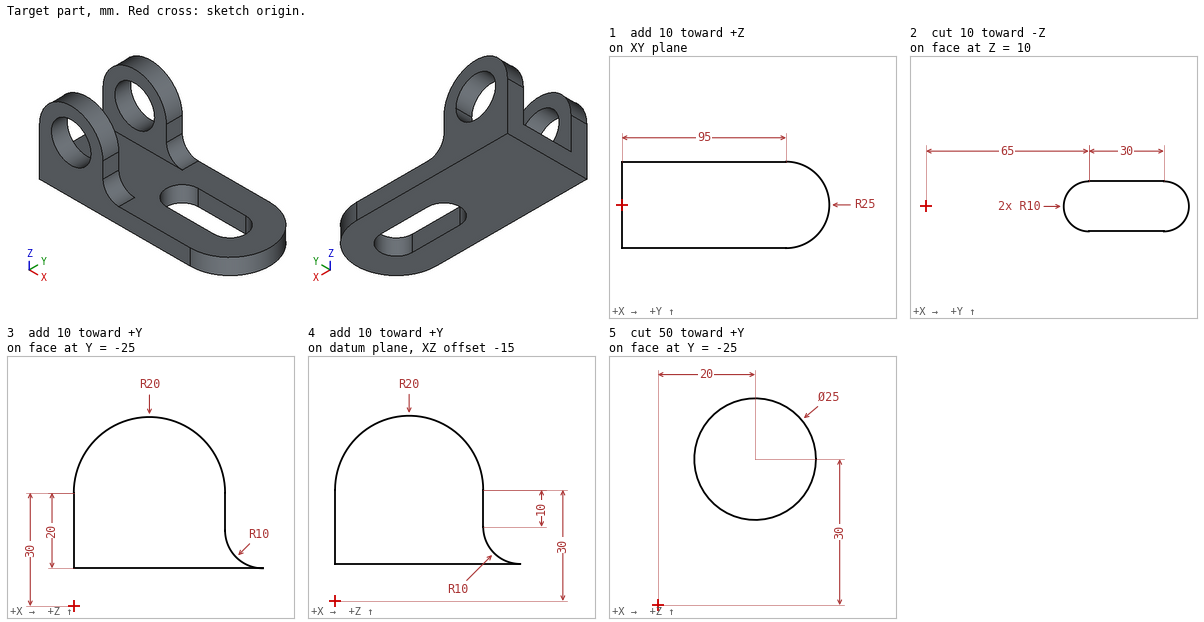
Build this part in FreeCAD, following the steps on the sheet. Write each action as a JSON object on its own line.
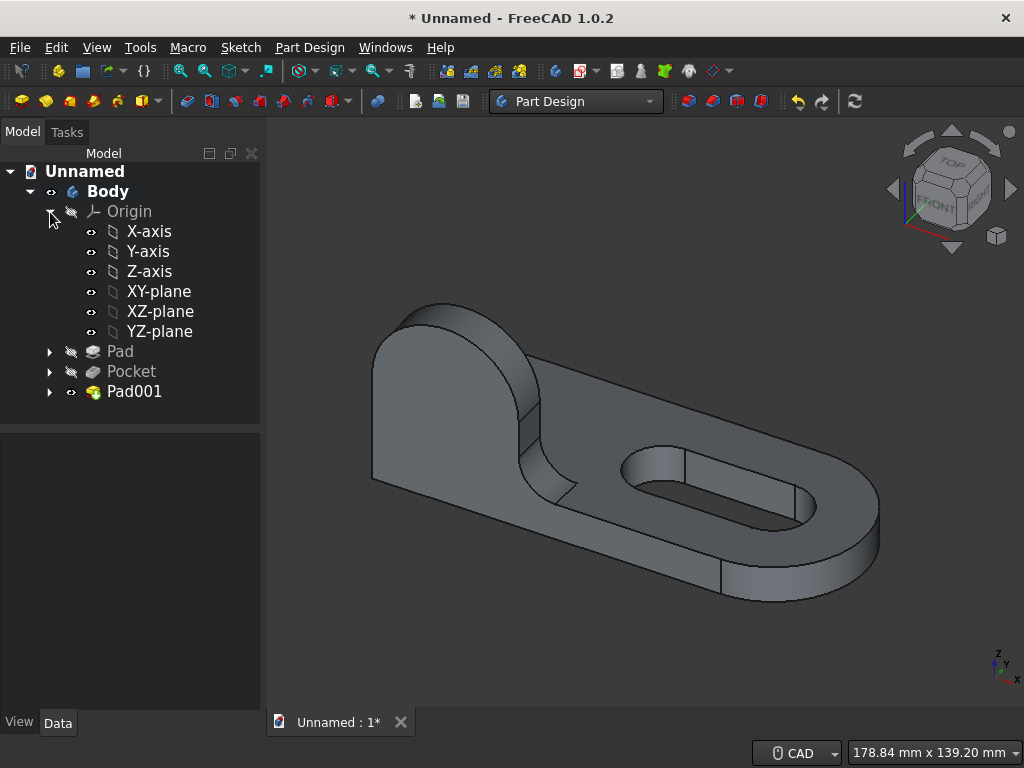
{"action": "left_click", "coordinate": [136, 312]}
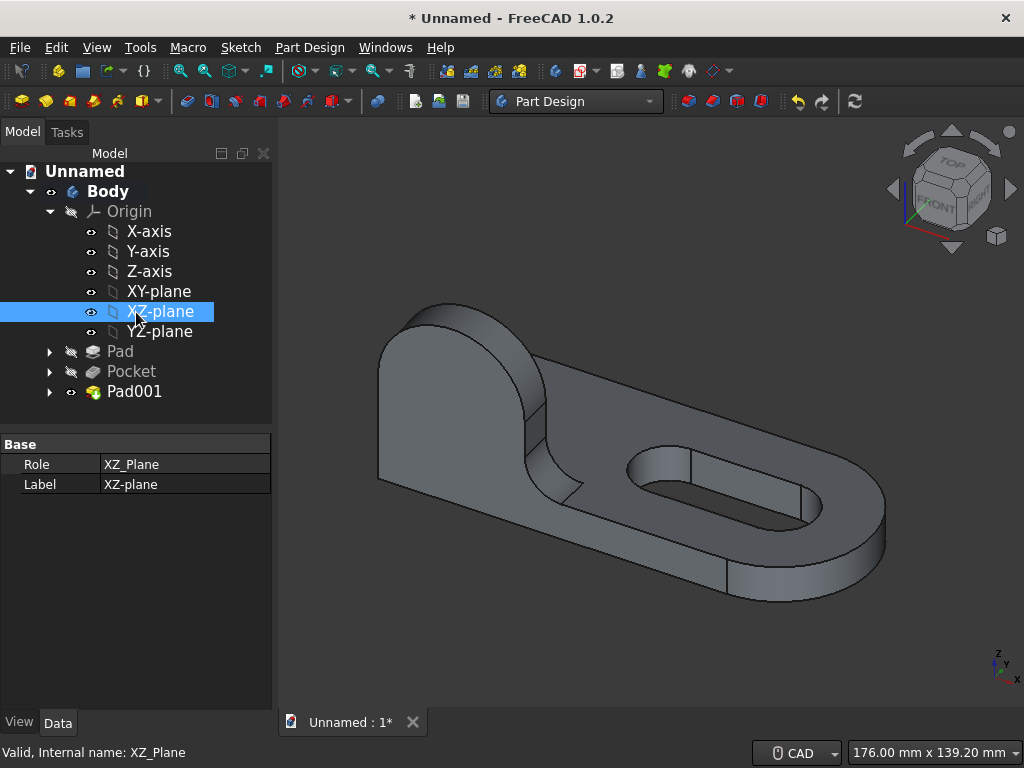
{"action": "left_click", "coordinate": [714, 72]}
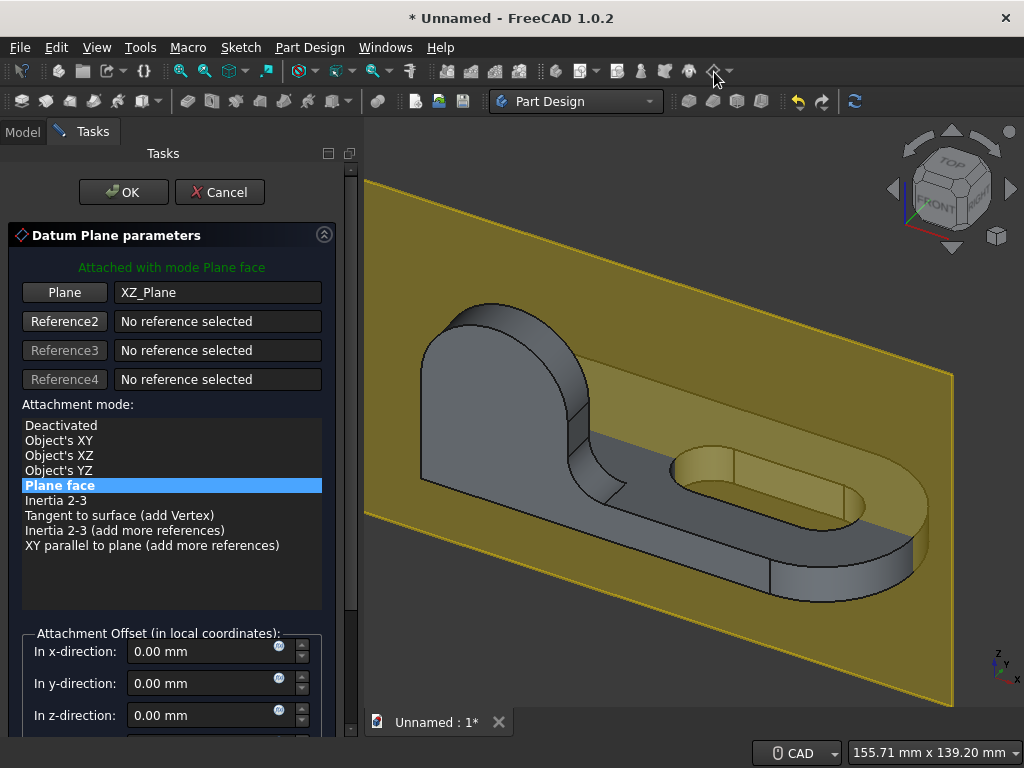
{"action": "triple_click", "coordinate": [210, 715]}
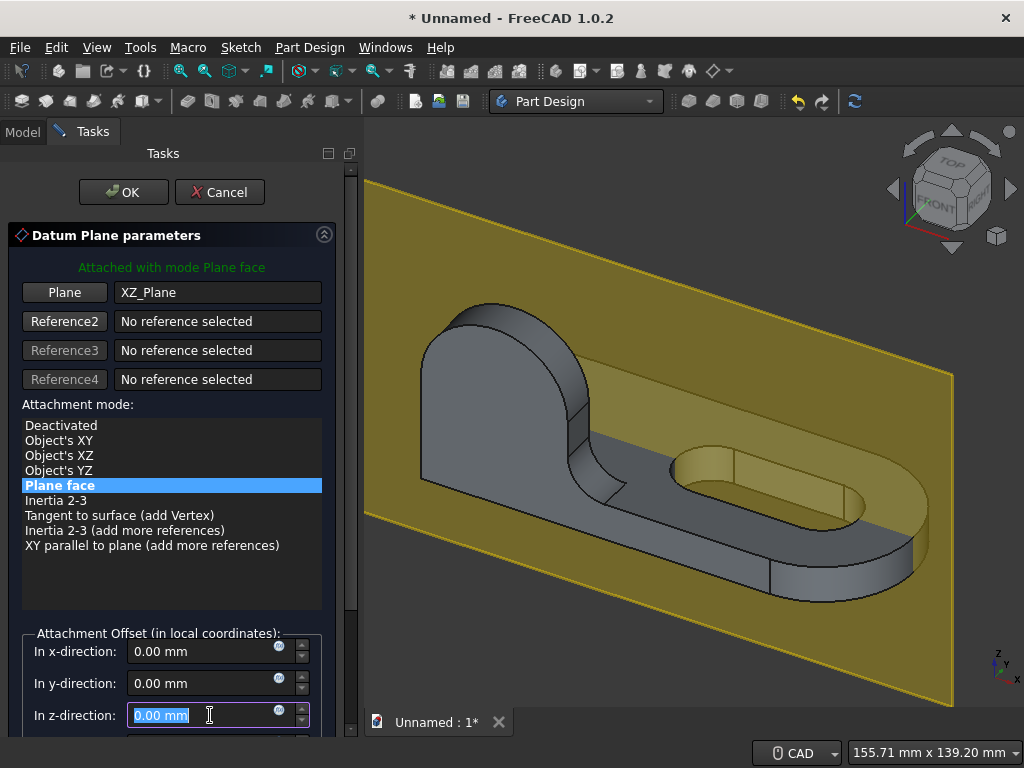
{"action": "type", "text": "-15"}
{"action": "key", "text": "Tab"}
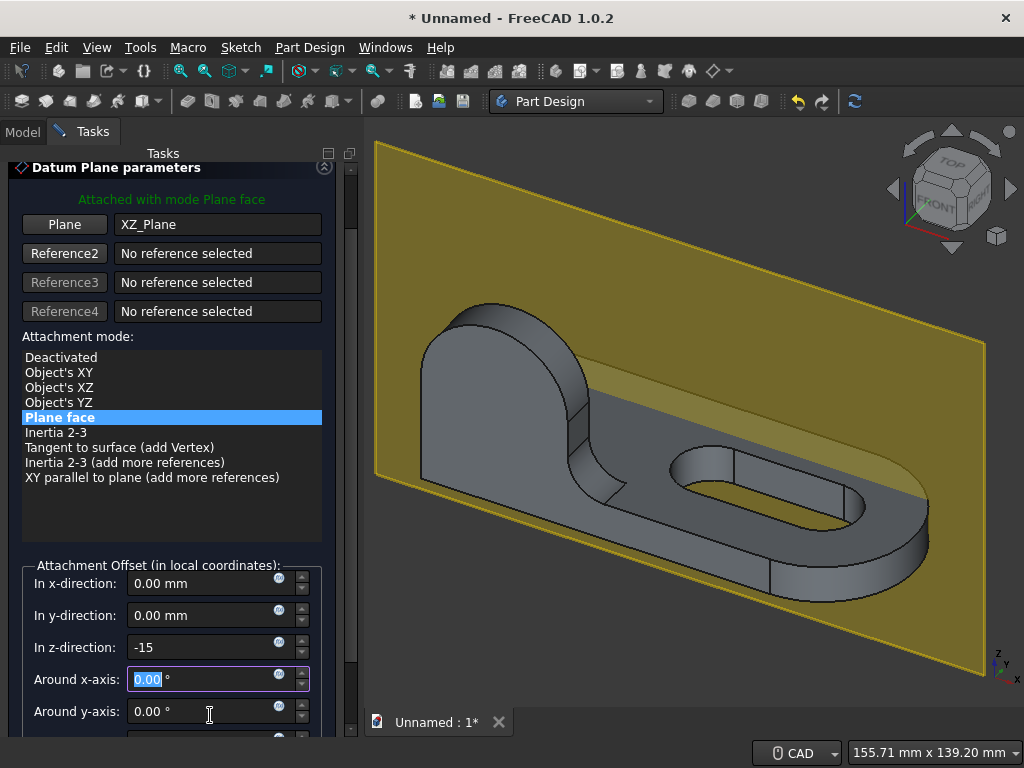
{"action": "scroll", "coordinate": [351, 450], "scroll_direction": "up", "scroll_amount": 2}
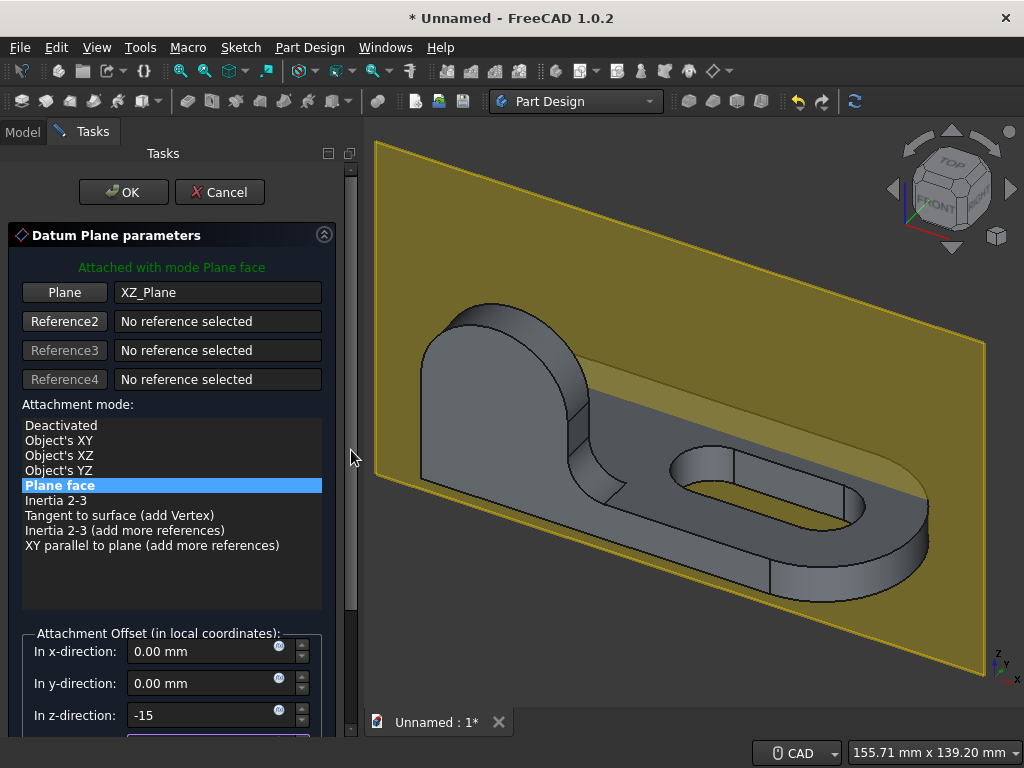
{"action": "left_click", "coordinate": [124, 192]}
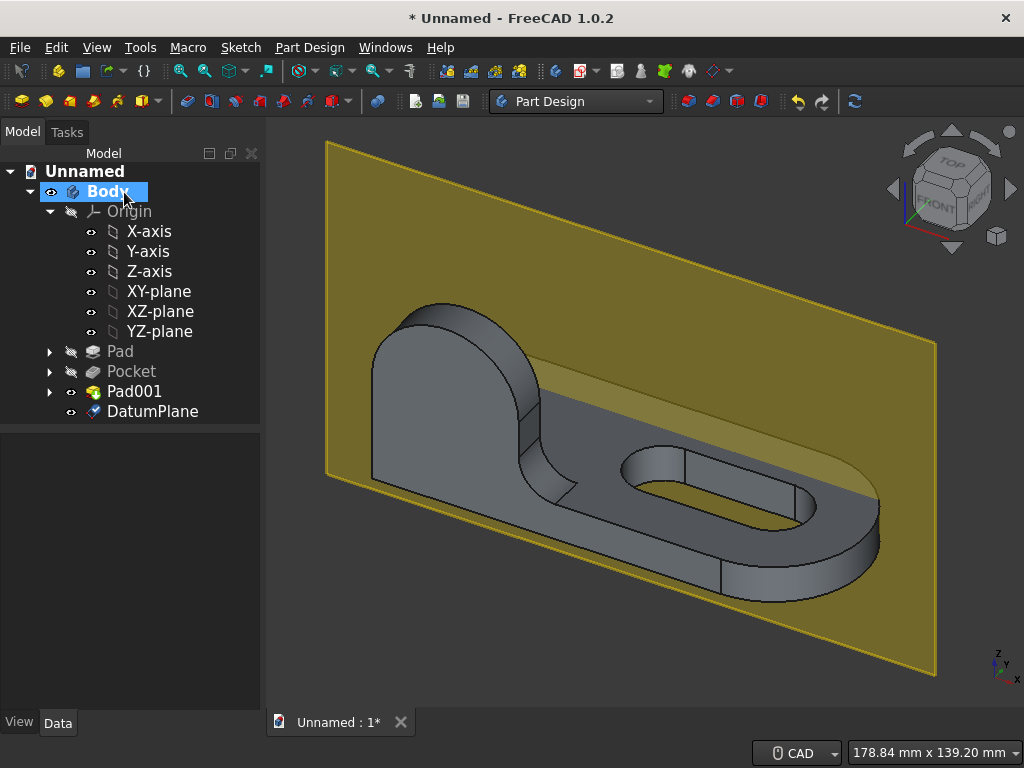
{"action": "left_click", "coordinate": [116, 412]}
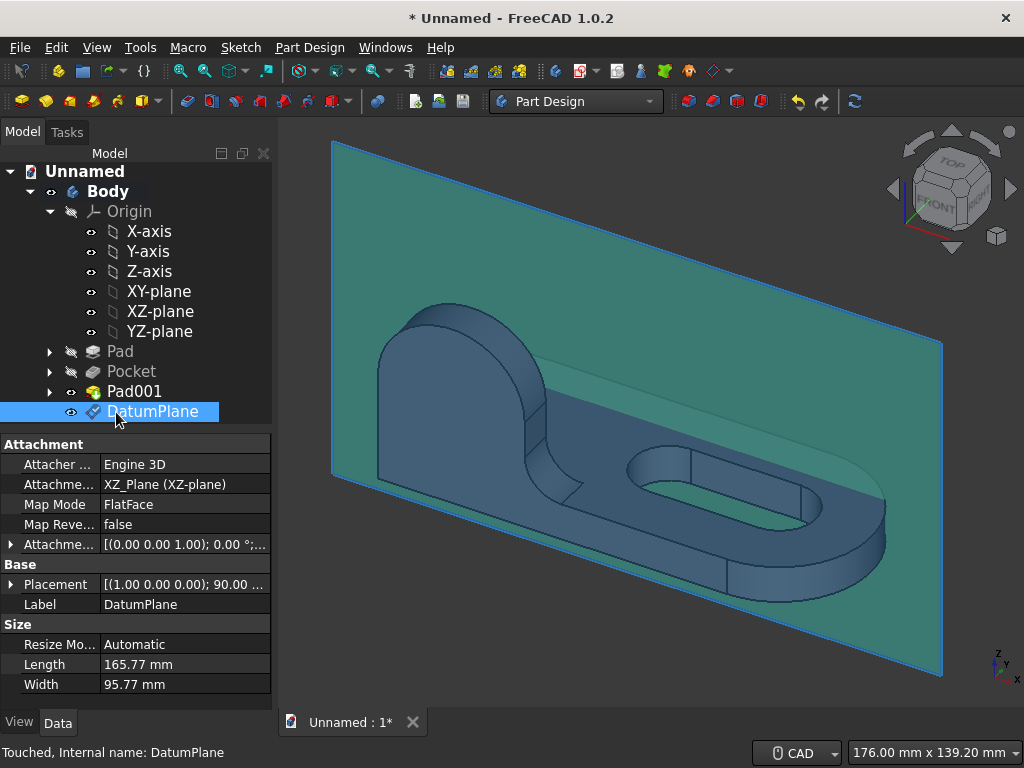
{"action": "left_click", "coordinate": [580, 72]}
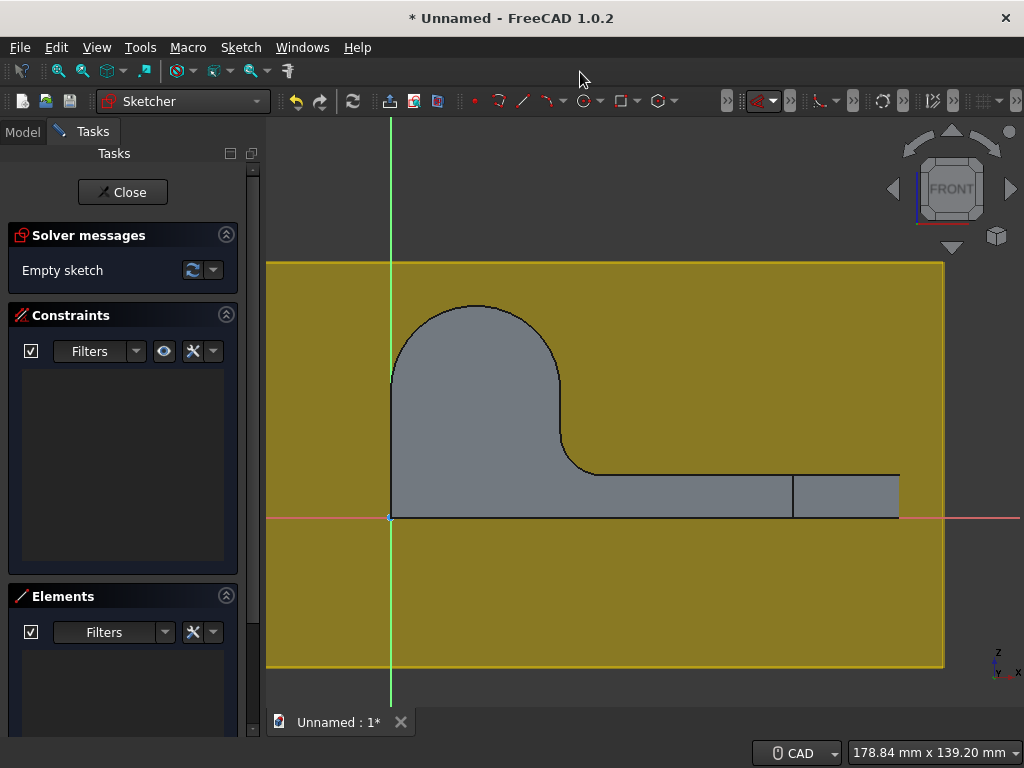
{"action": "left_click", "coordinate": [438, 102]}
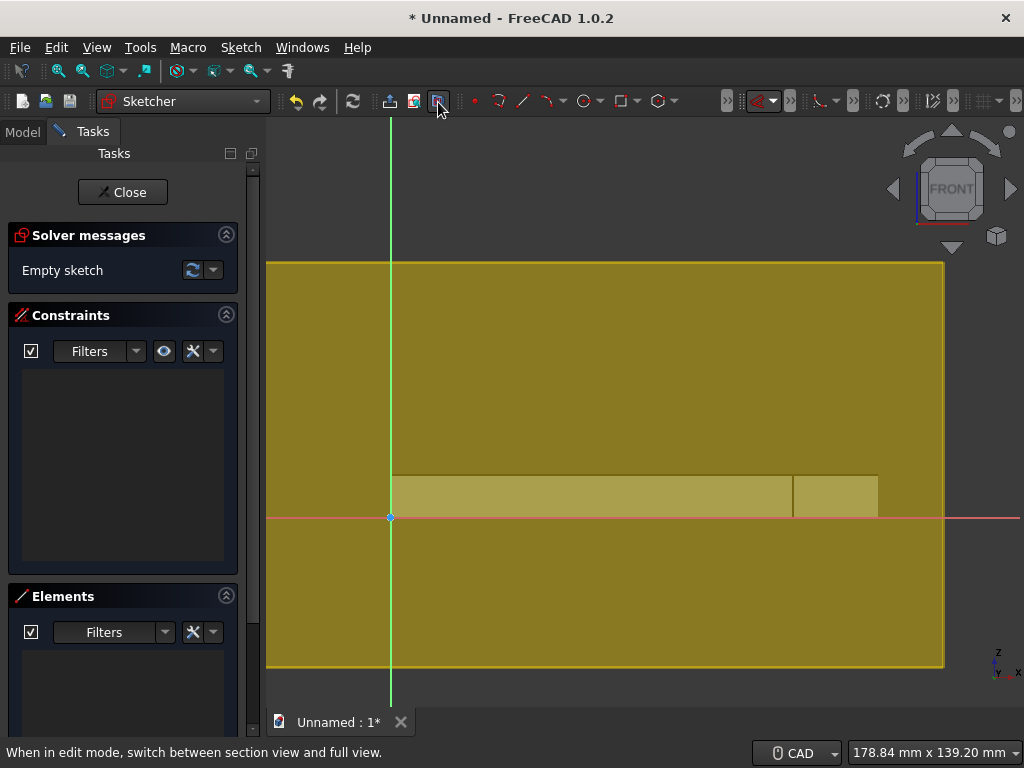
{"action": "scroll", "coordinate": [400, 412], "scroll_direction": "up", "scroll_amount": 3}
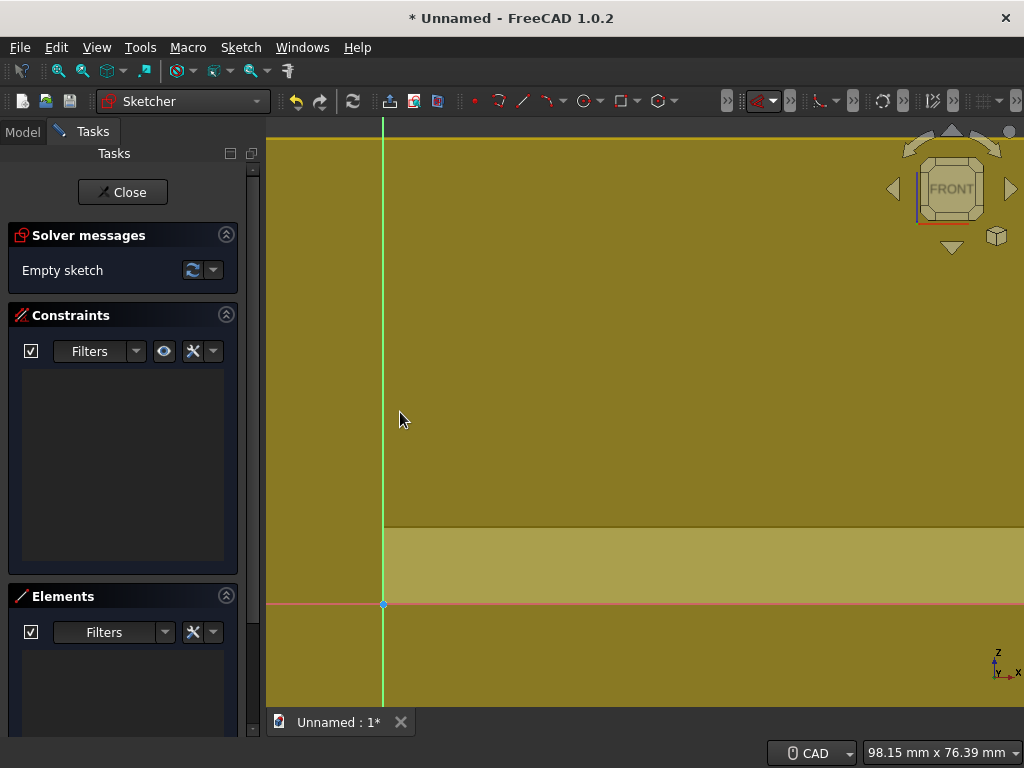
{"action": "left_click", "coordinate": [524, 102]}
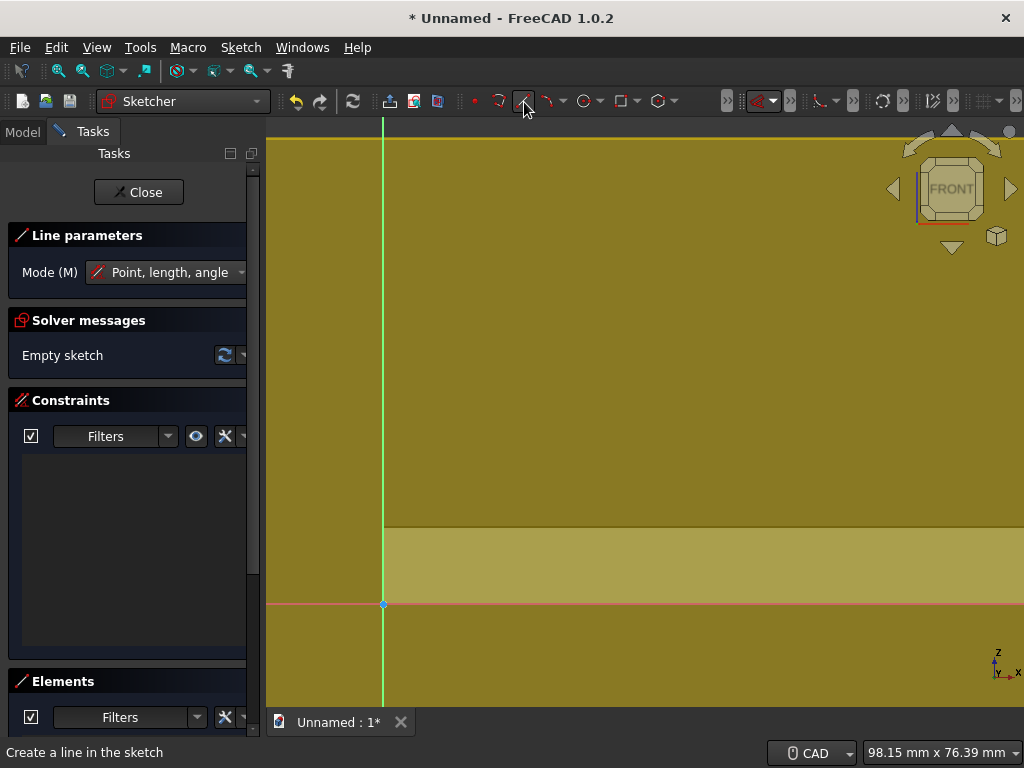
{"action": "left_click", "coordinate": [692, 373]}
{"action": "left_click", "coordinate": [692, 450]}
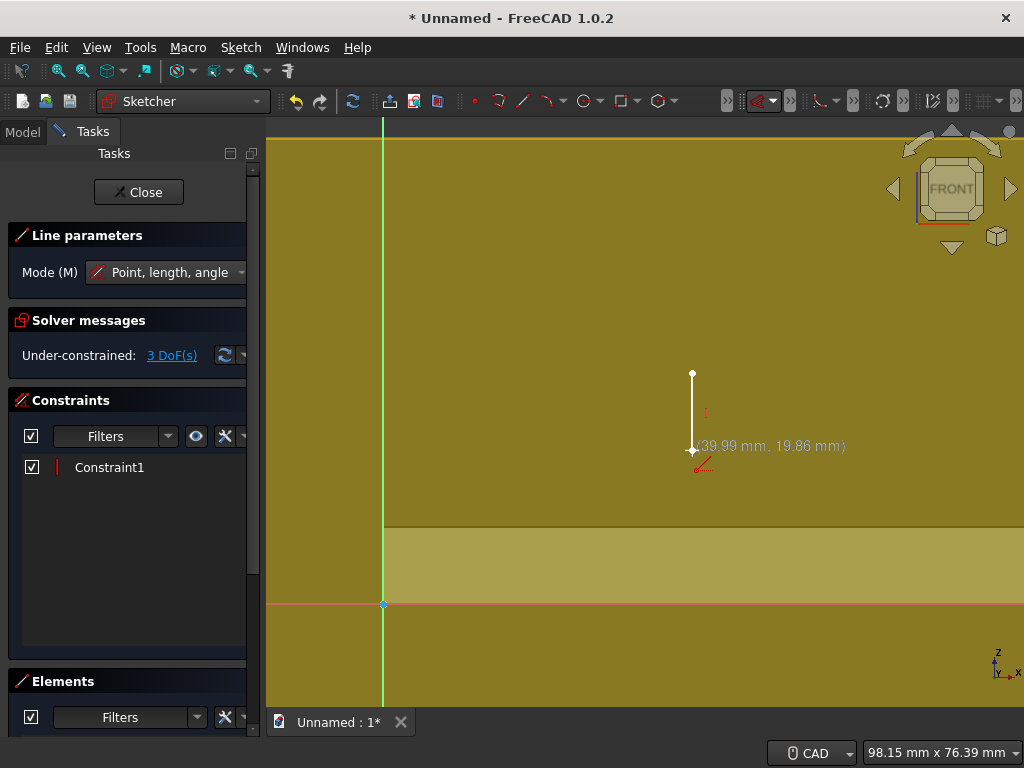
{"action": "left_click", "coordinate": [500, 102]}